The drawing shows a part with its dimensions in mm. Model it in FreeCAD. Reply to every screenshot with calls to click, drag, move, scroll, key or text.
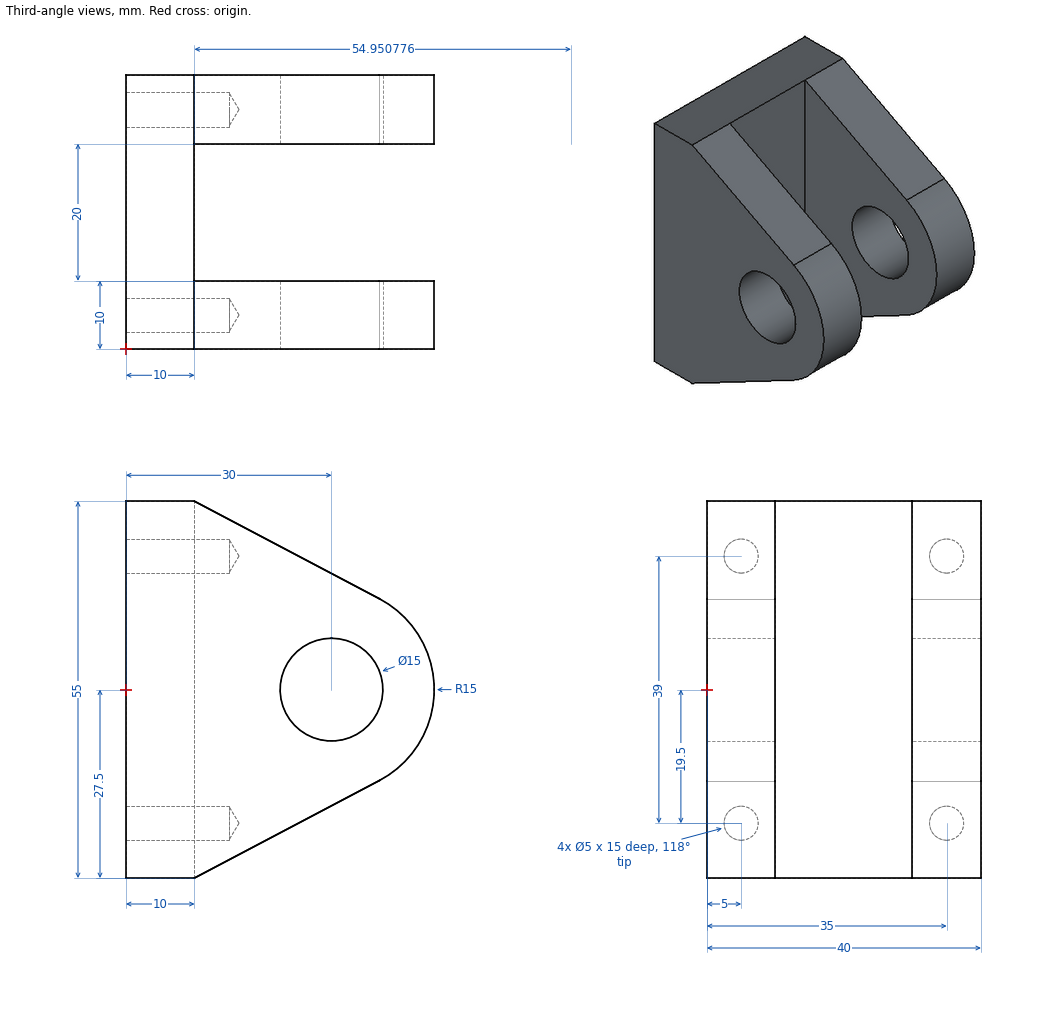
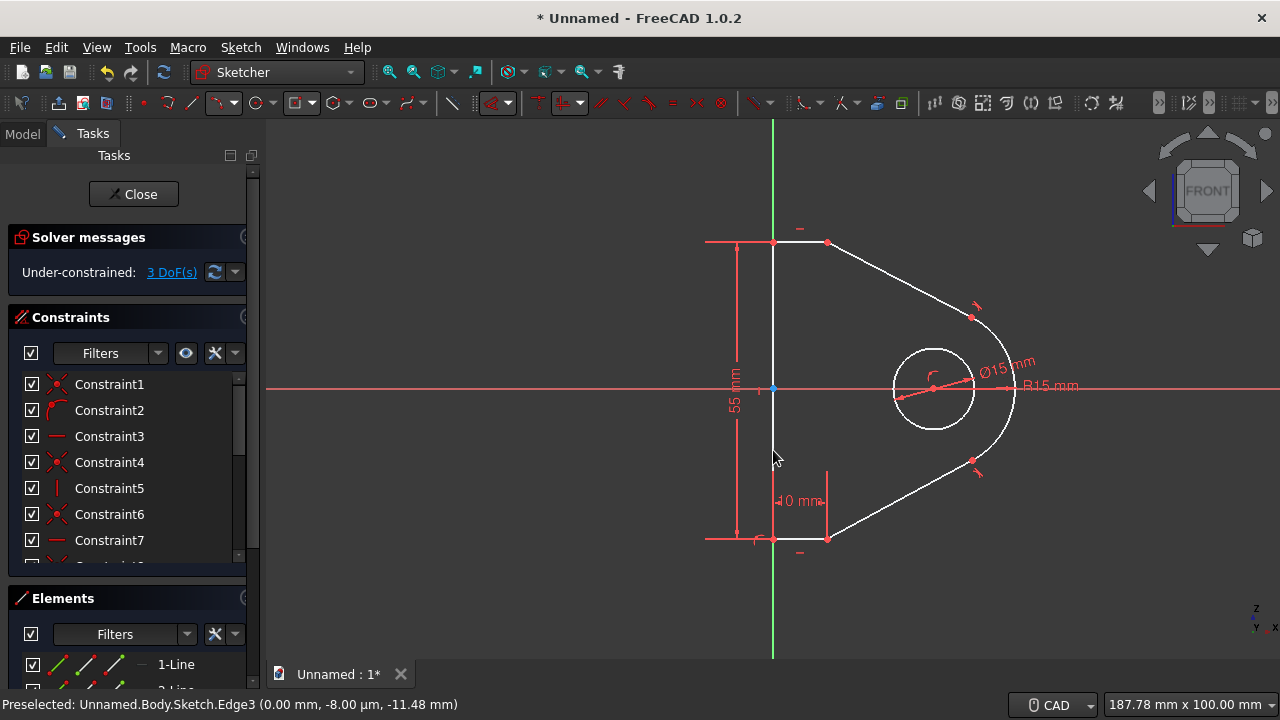
click(789, 242)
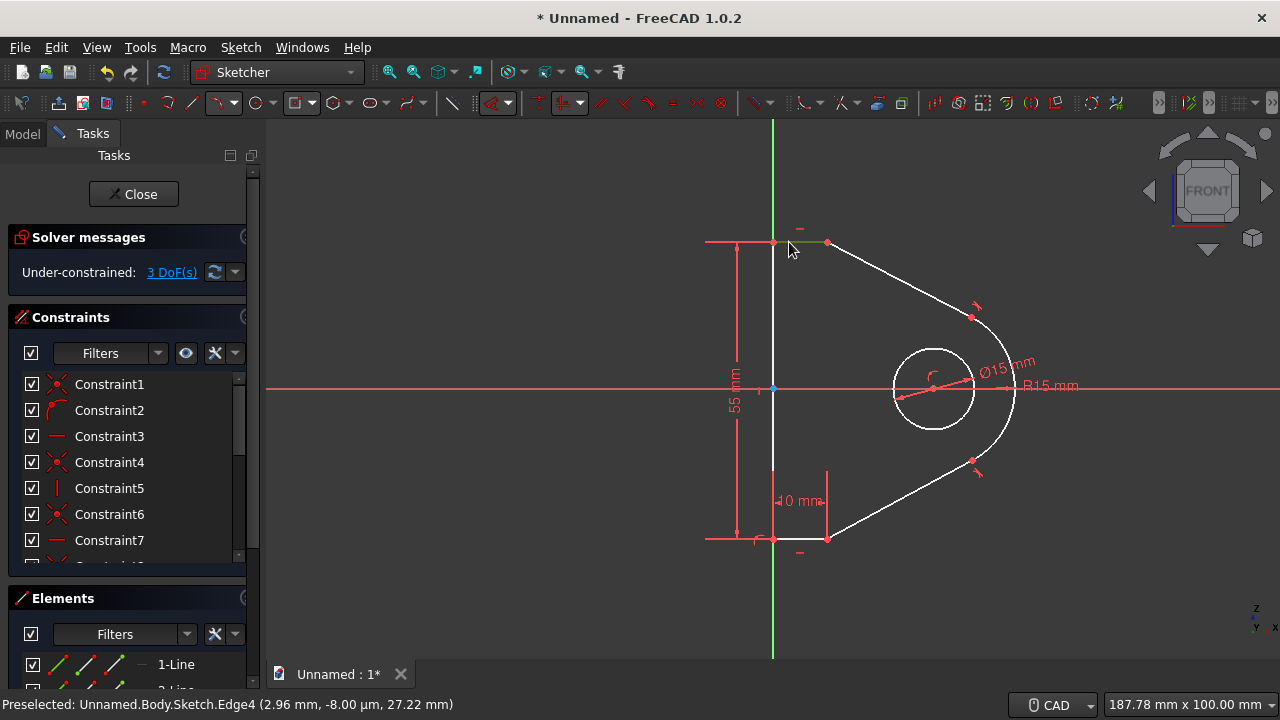
key(l)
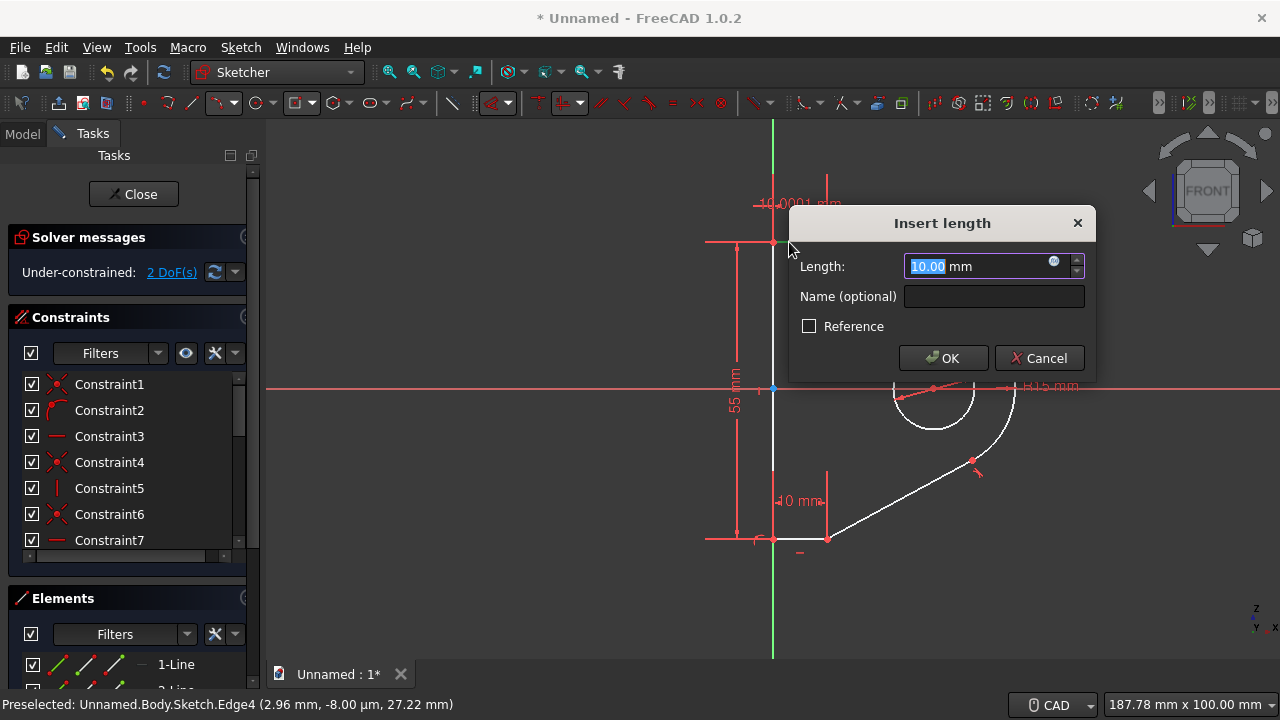
text(10)
key(Return)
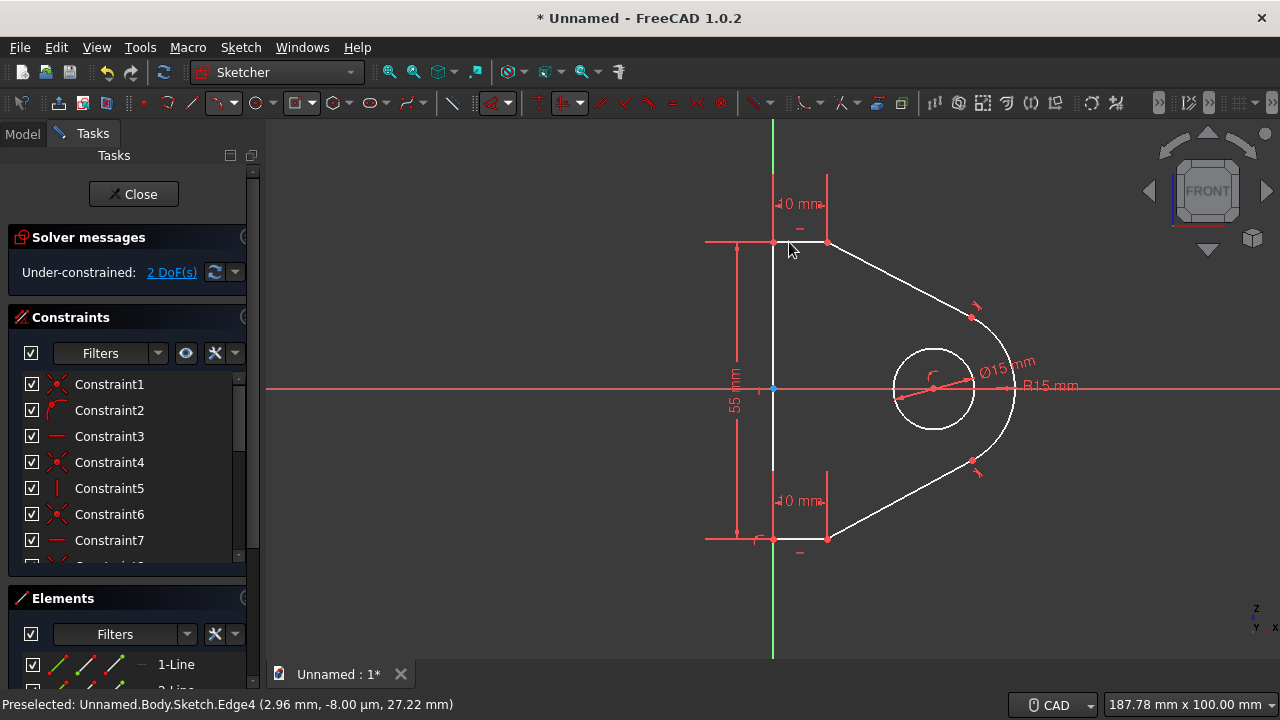
click(934, 389)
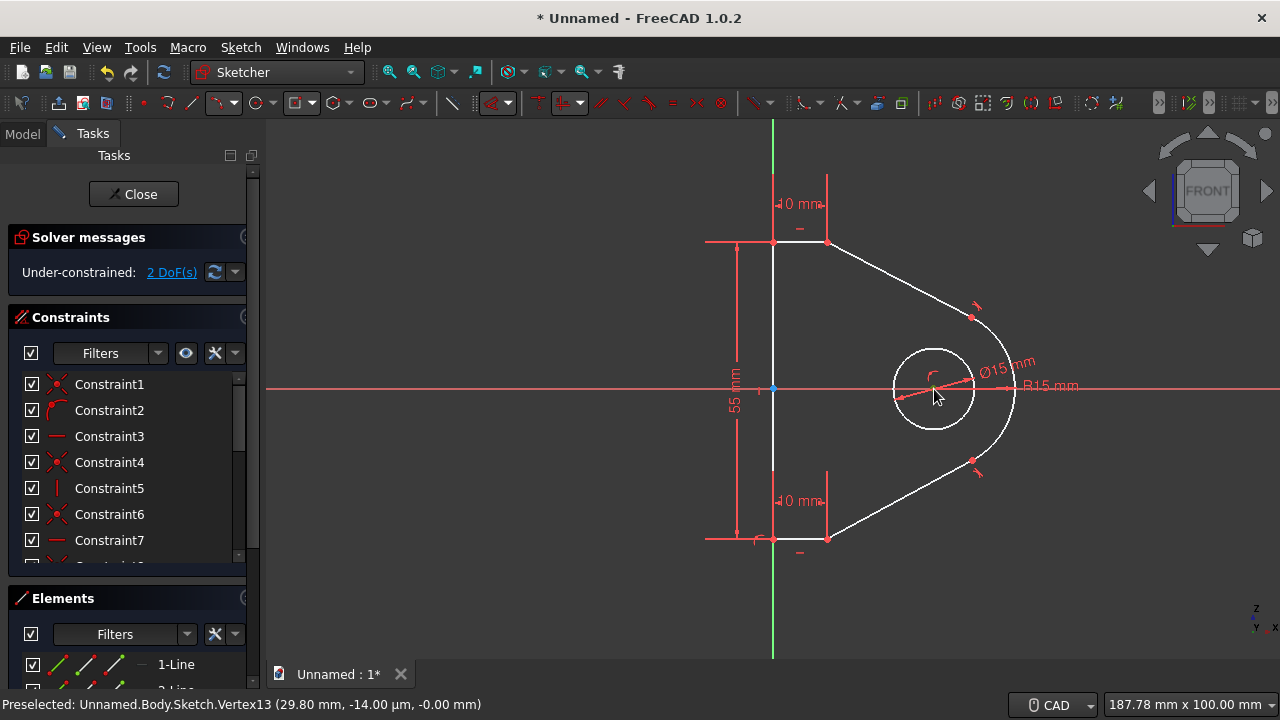
key(l)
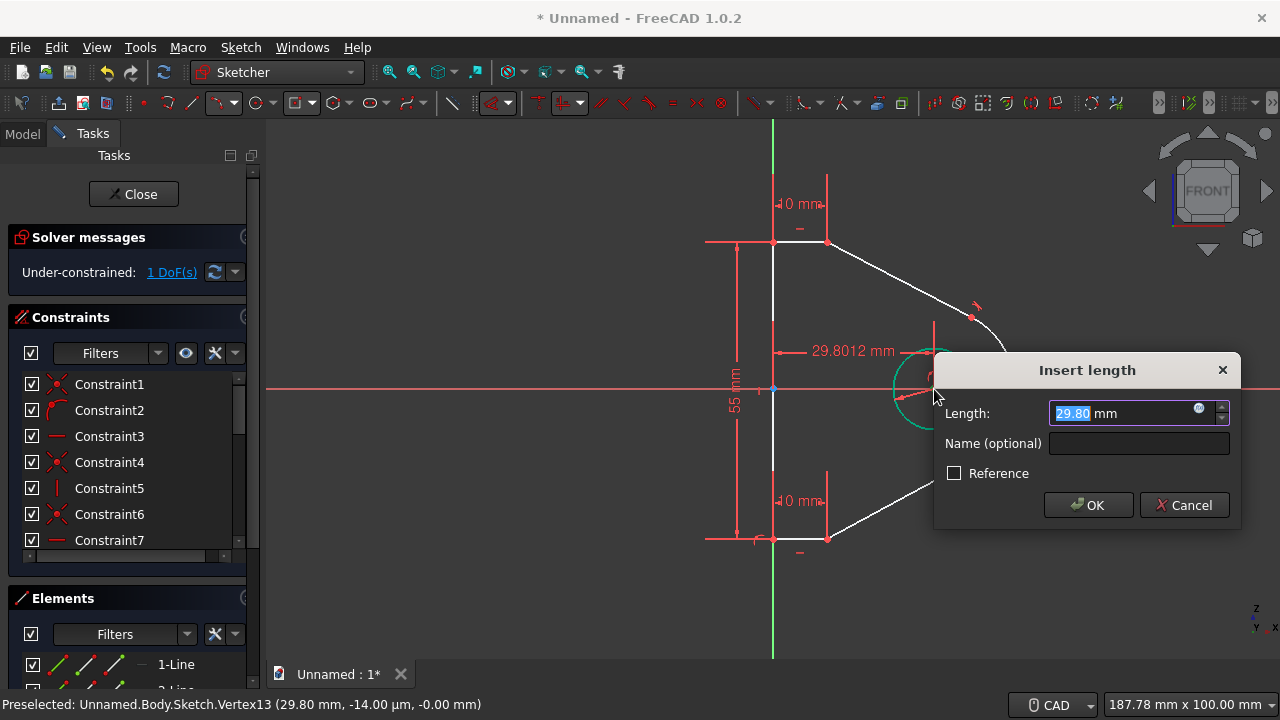
text(30)
key(Return)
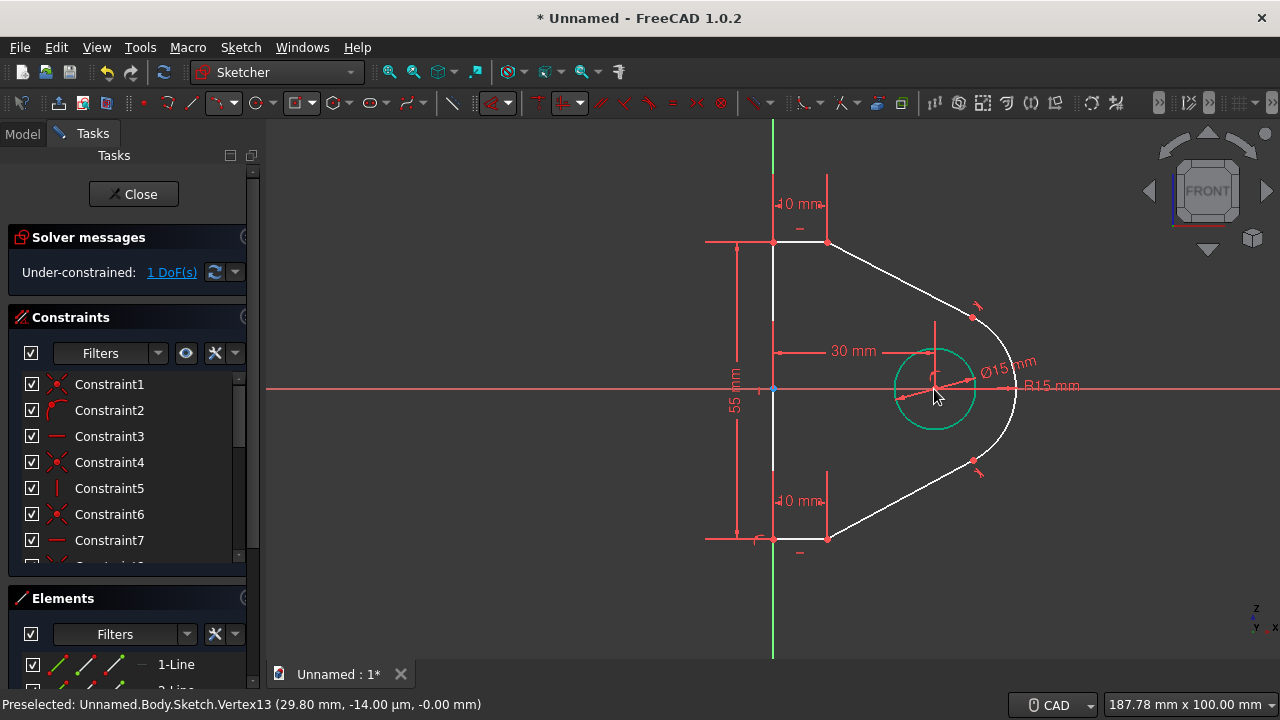
click(827, 539)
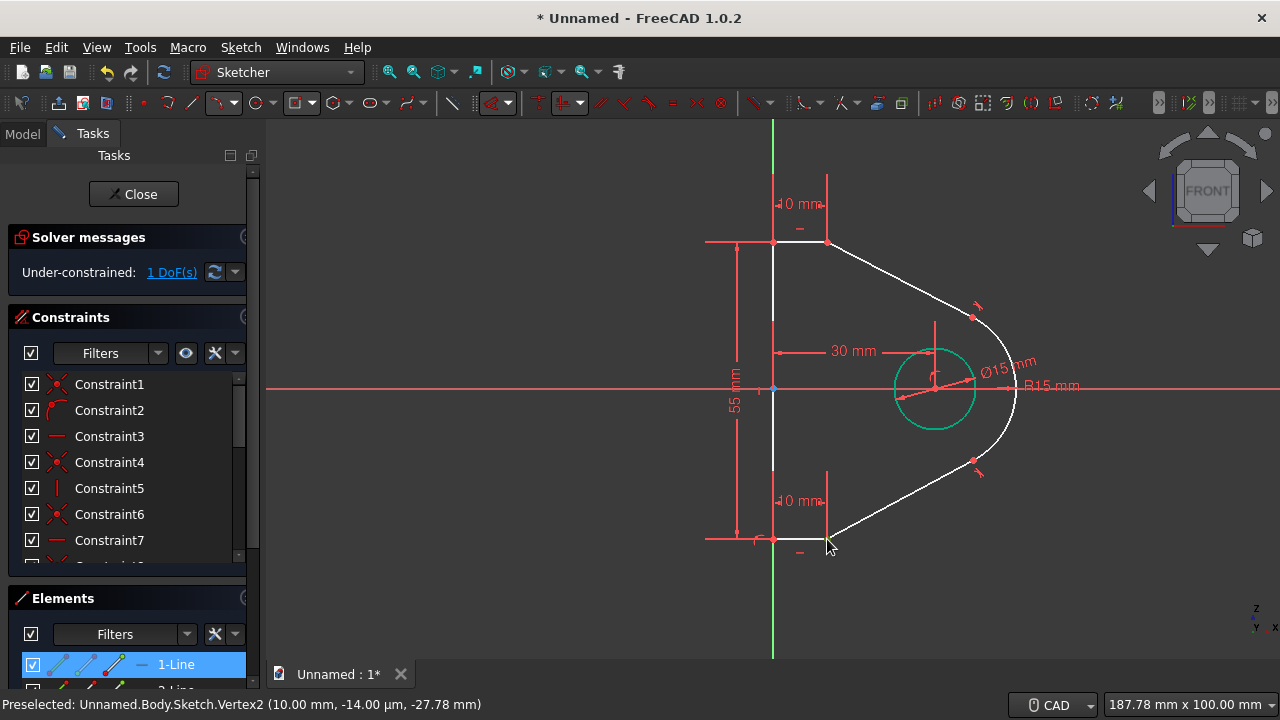
key(i)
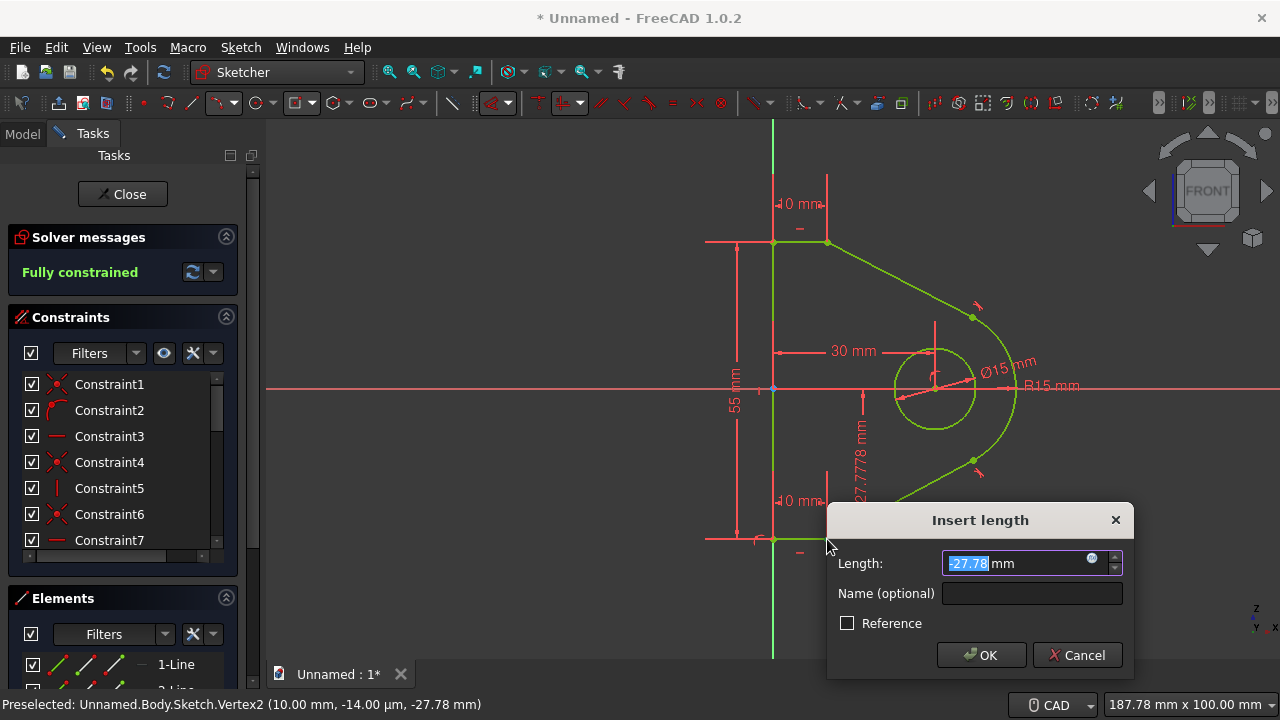
text(-27.5)
key(Return)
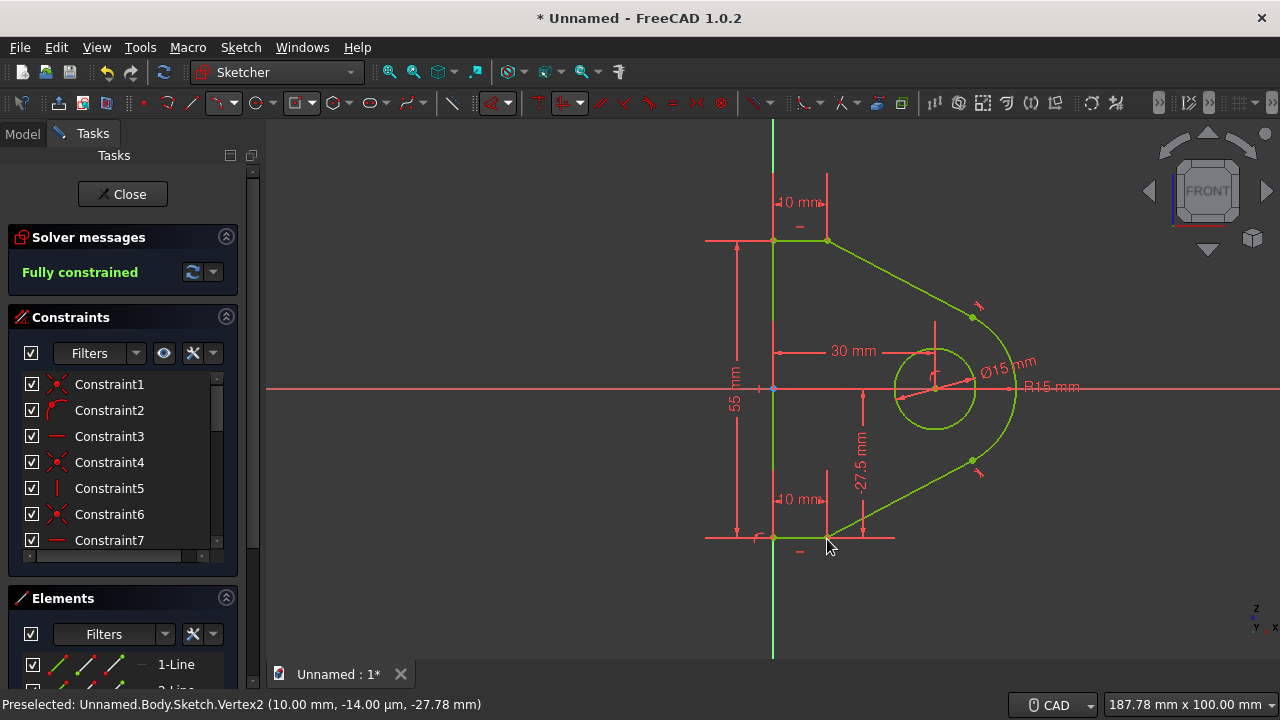
click(123, 194)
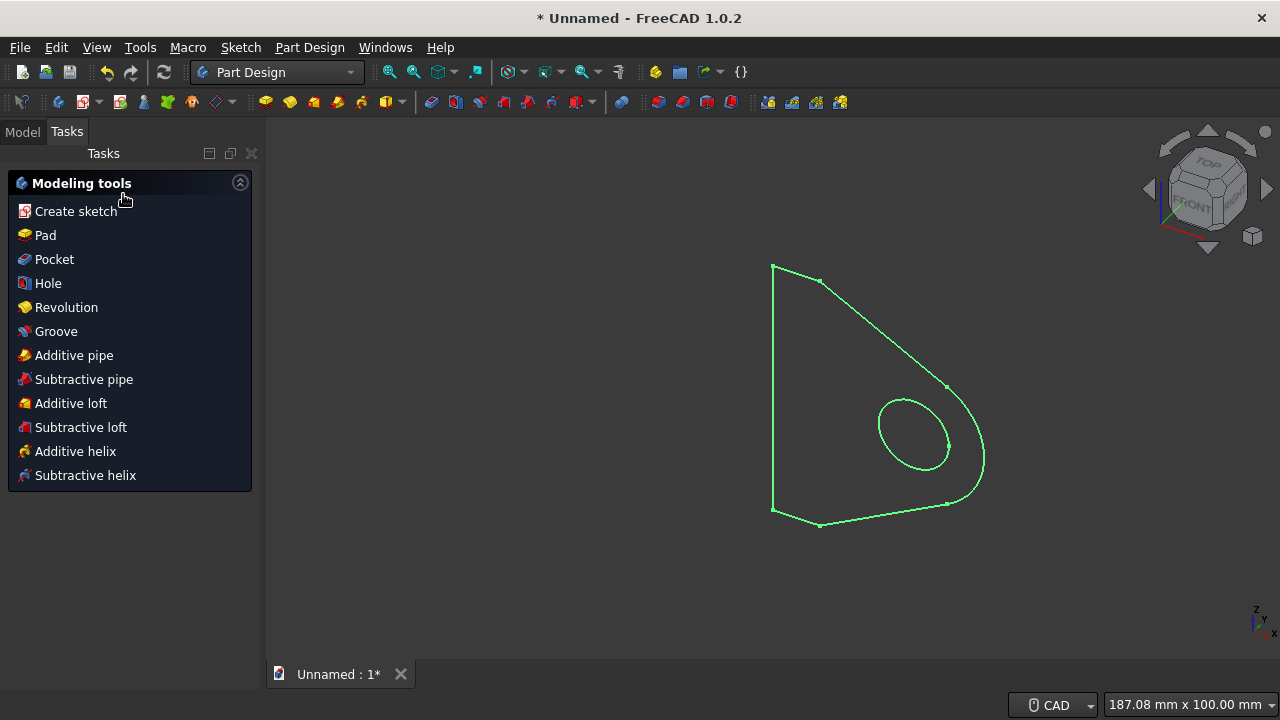
click(266, 102)